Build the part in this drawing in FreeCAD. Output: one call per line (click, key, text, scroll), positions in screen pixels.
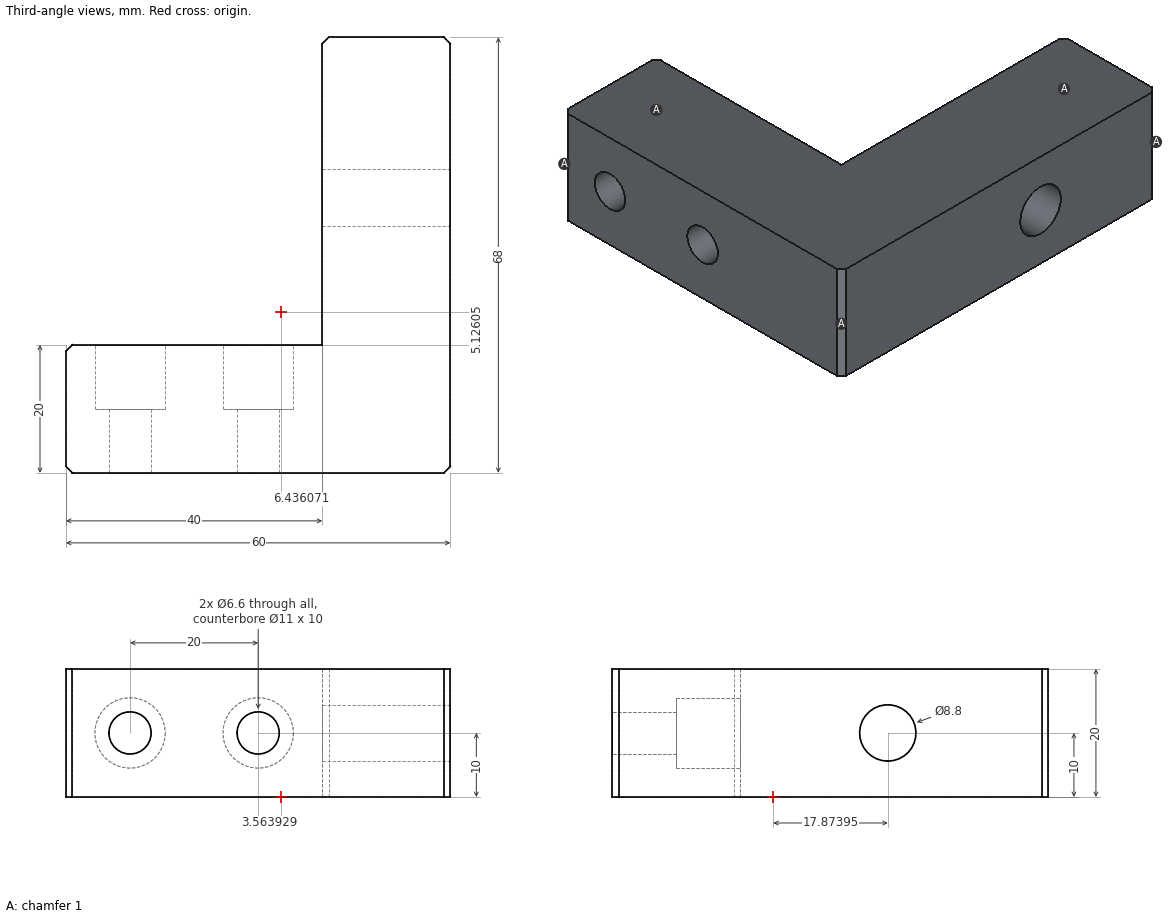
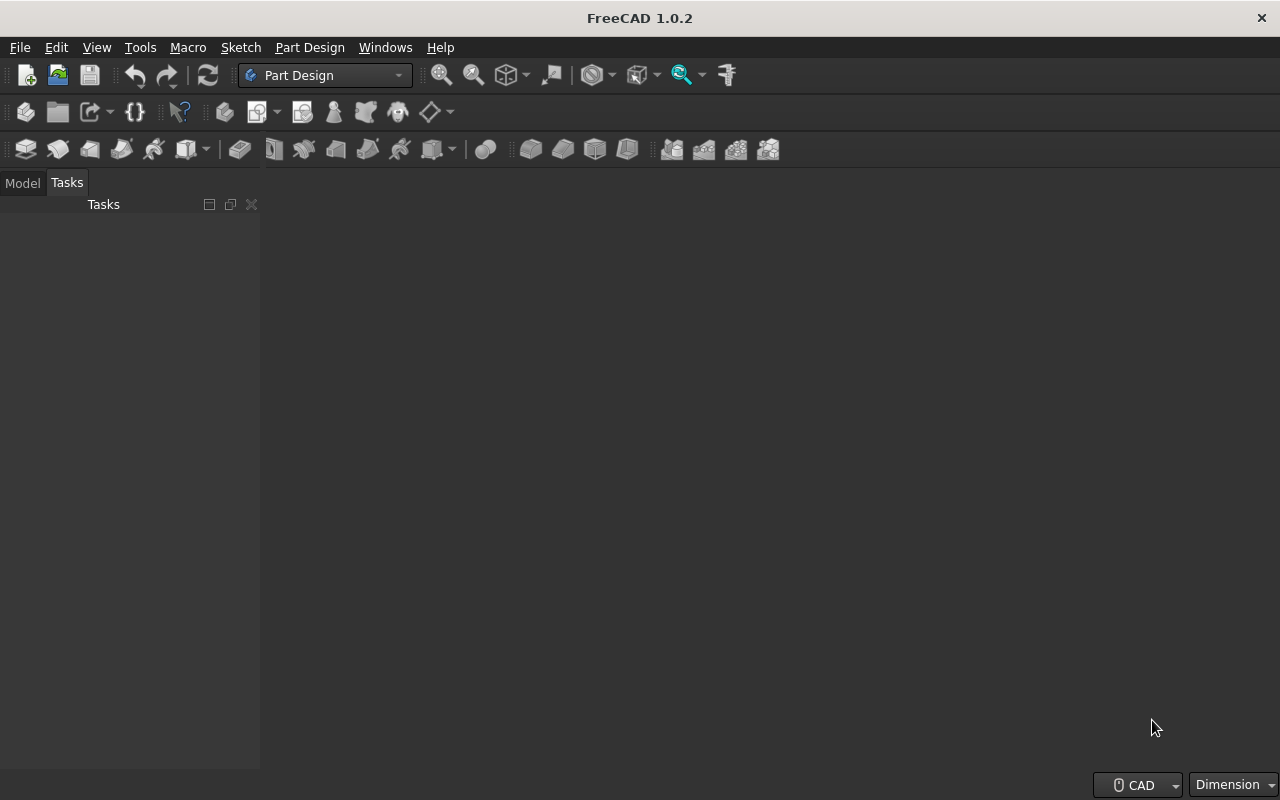
click(26, 76)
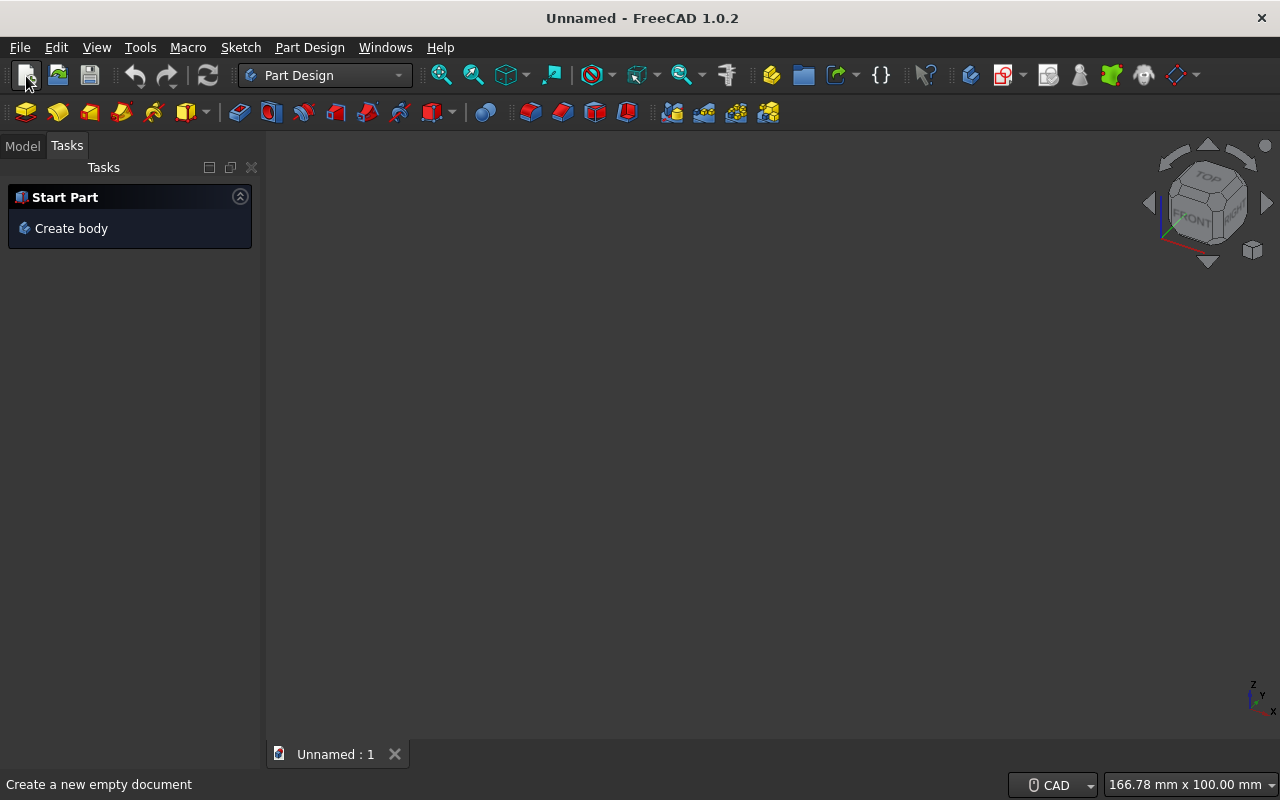
click(1004, 76)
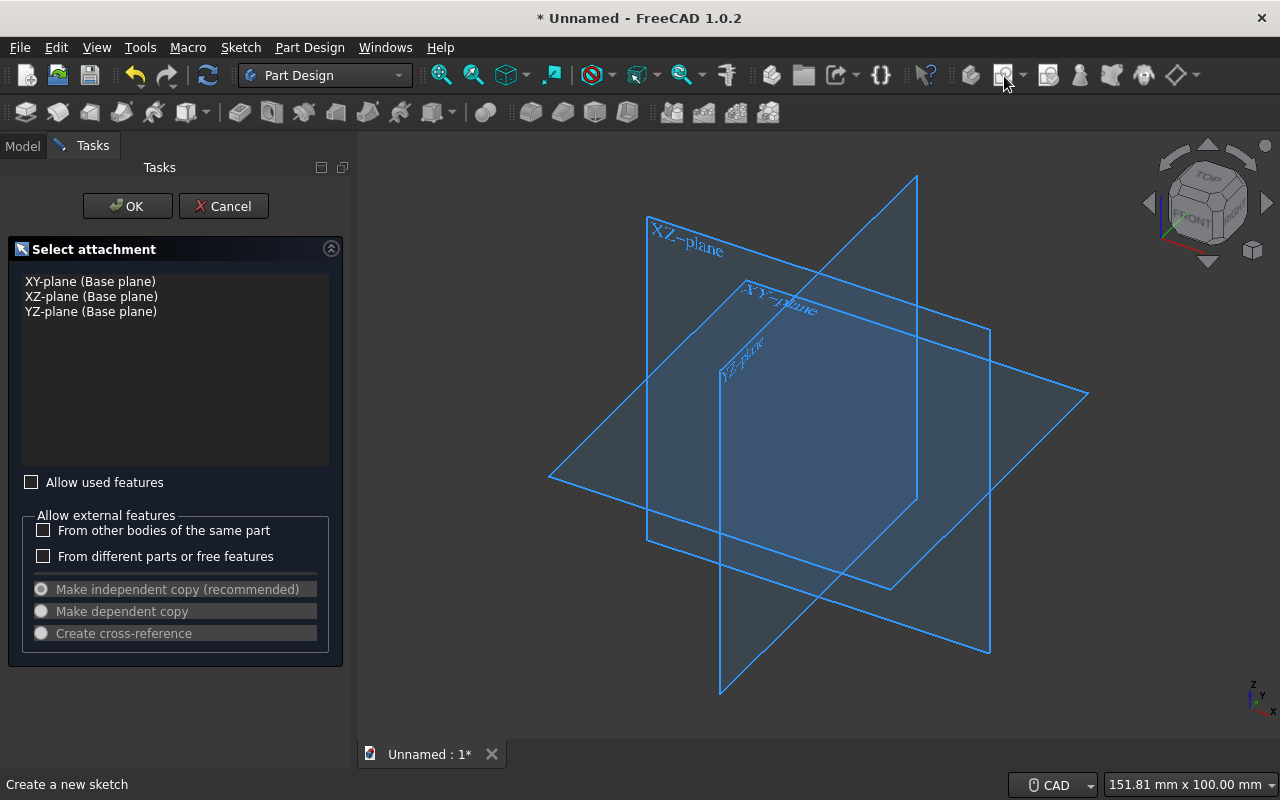
click(82, 282)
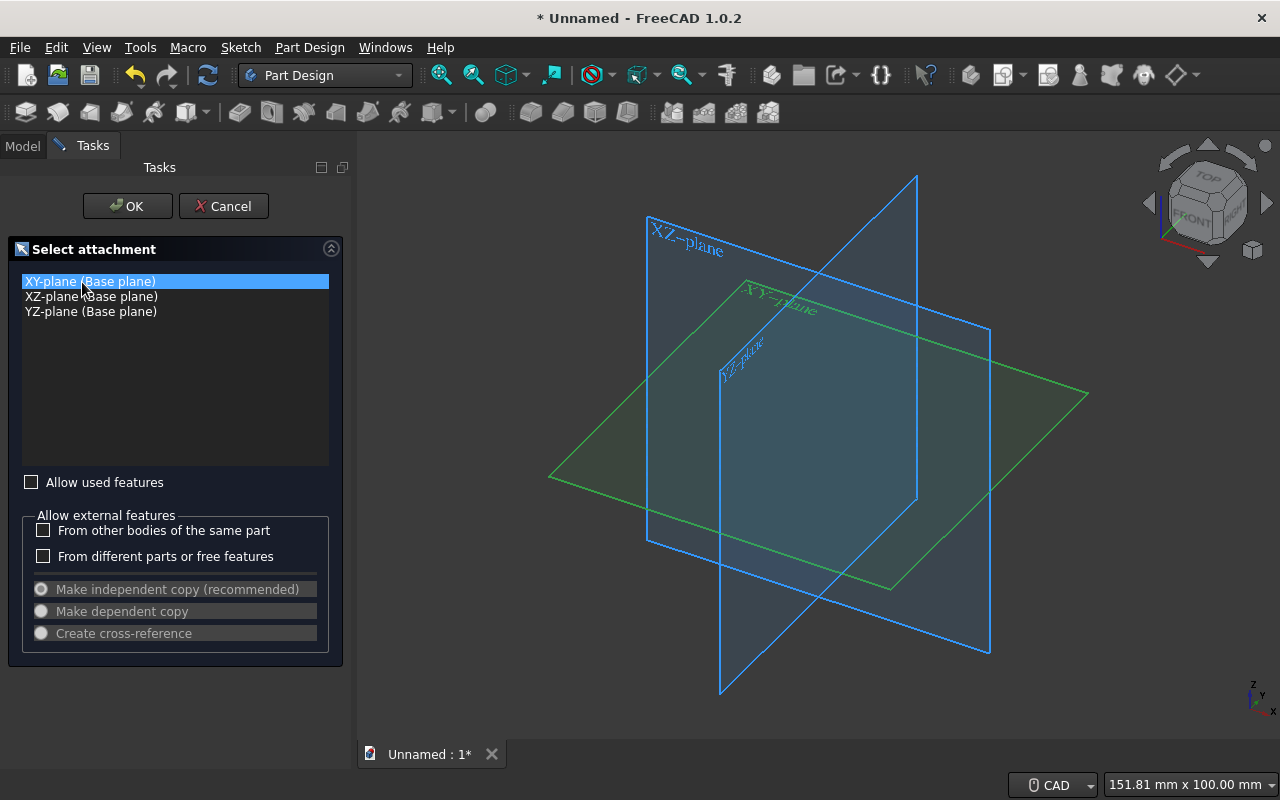
click(128, 206)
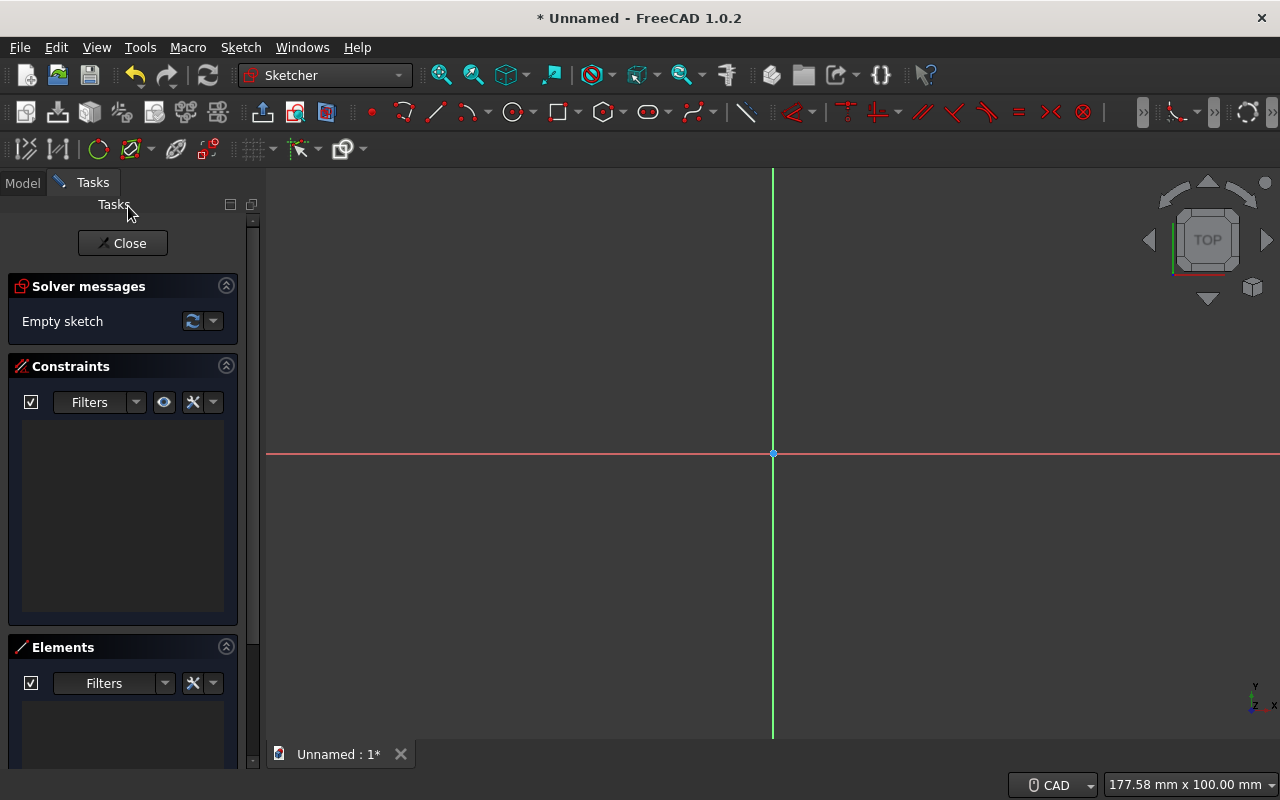
scroll(487, 682, down, 1)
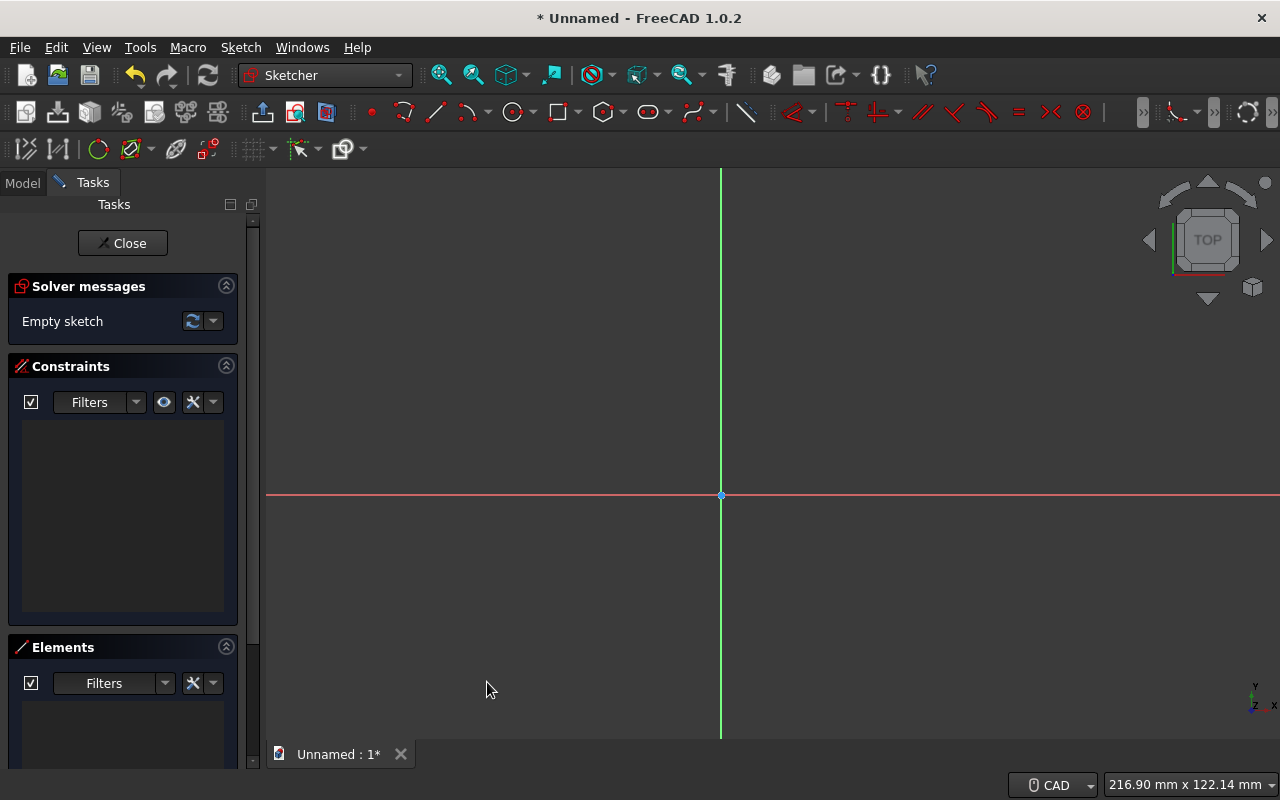
click(404, 112)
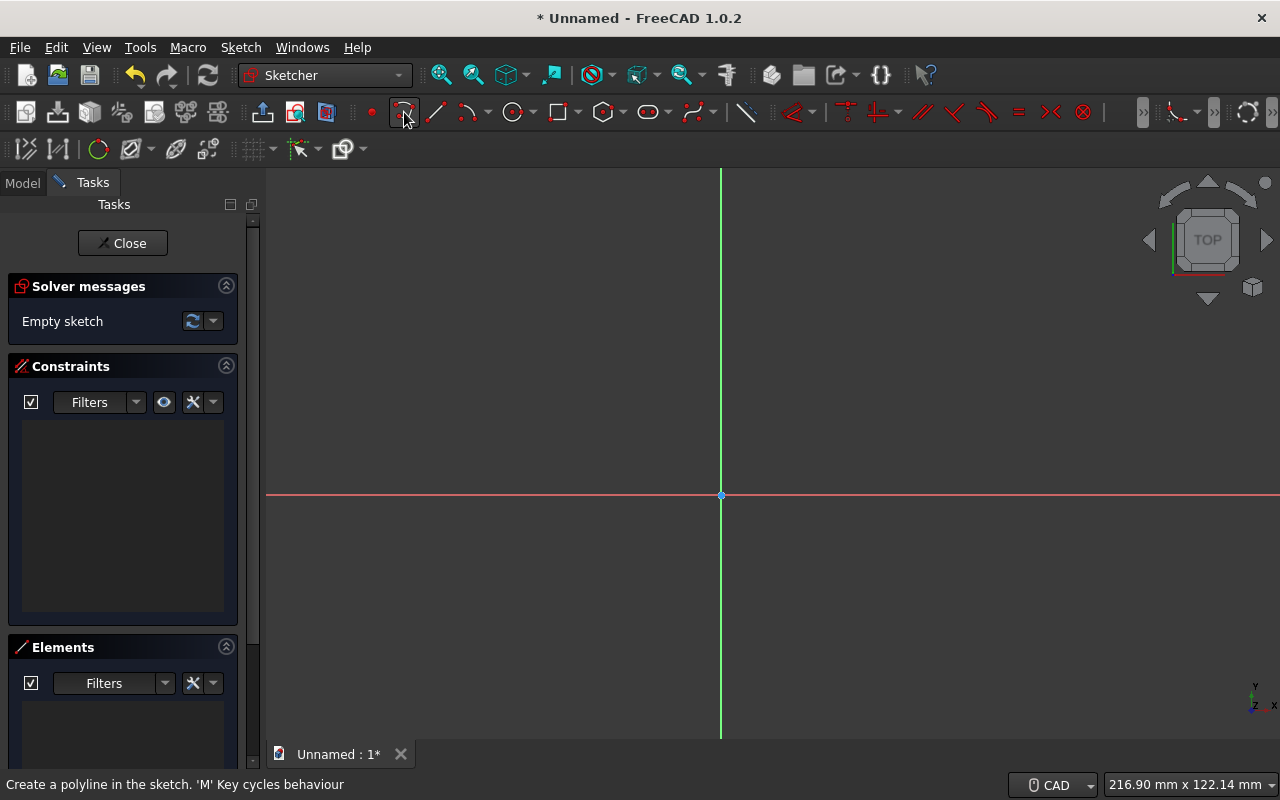
click(751, 519)
click(564, 519)
click(564, 613)
click(845, 613)
click(845, 295)
click(751, 295)
click(751, 520)
key(Escape)
key(Escape)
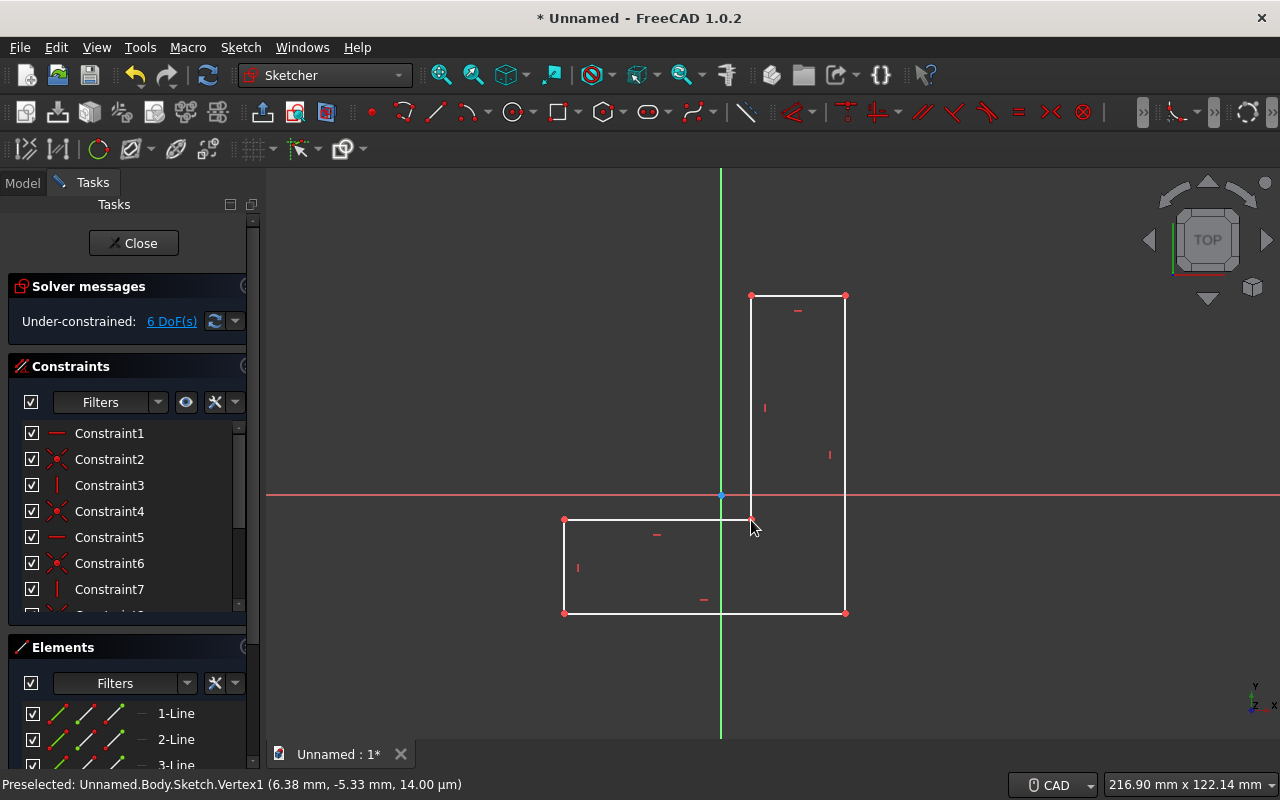
key(d)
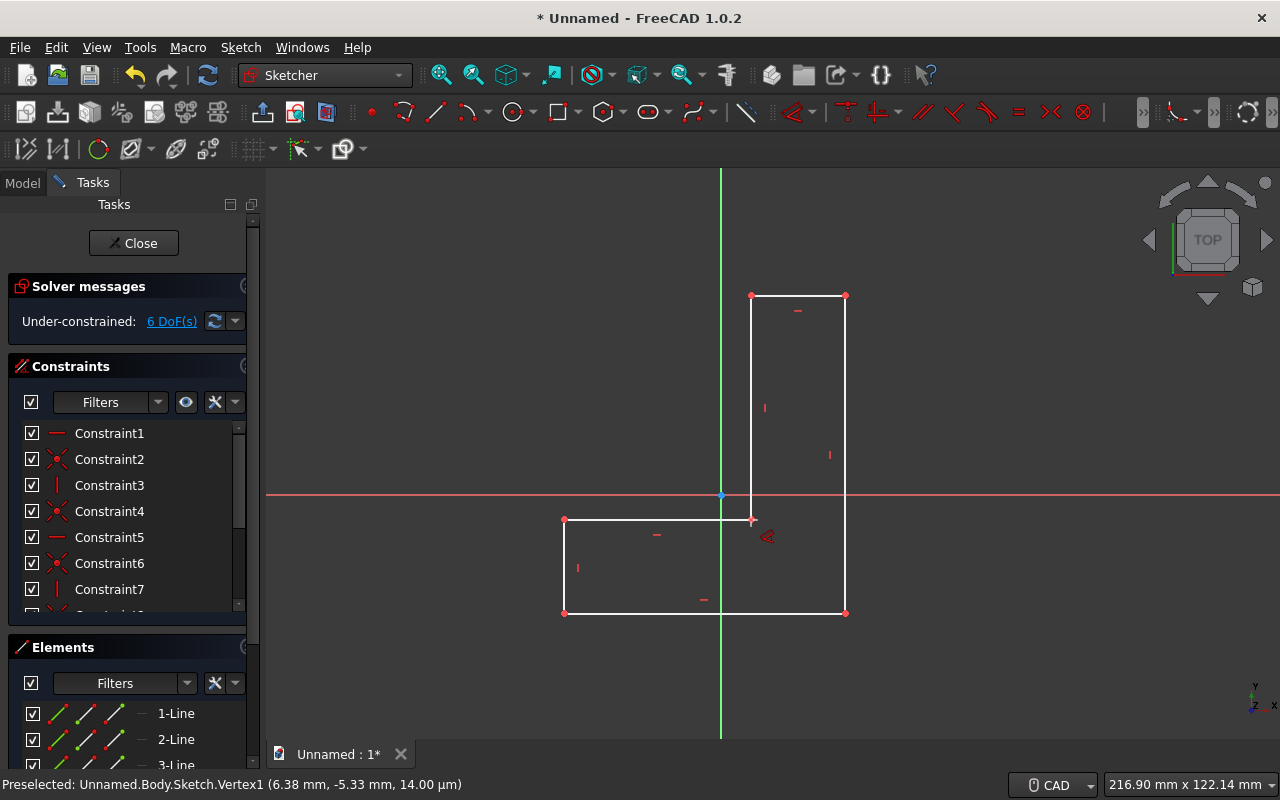
click(695, 520)
click(658, 554)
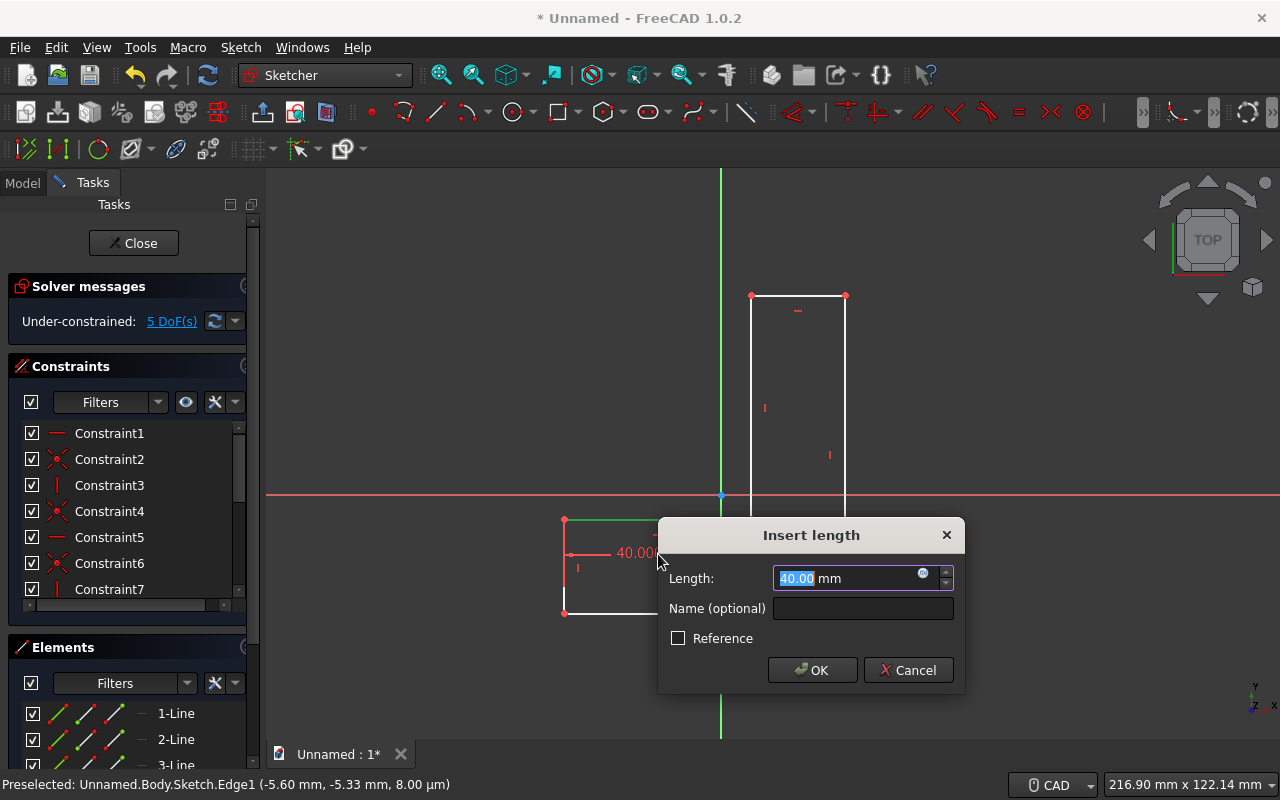
text(40)
key(Return)